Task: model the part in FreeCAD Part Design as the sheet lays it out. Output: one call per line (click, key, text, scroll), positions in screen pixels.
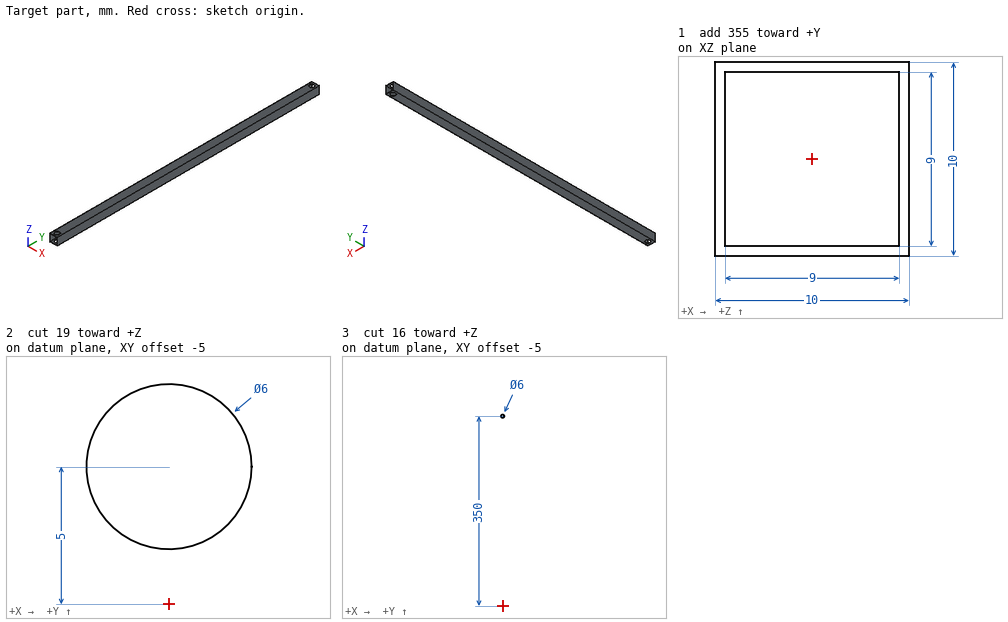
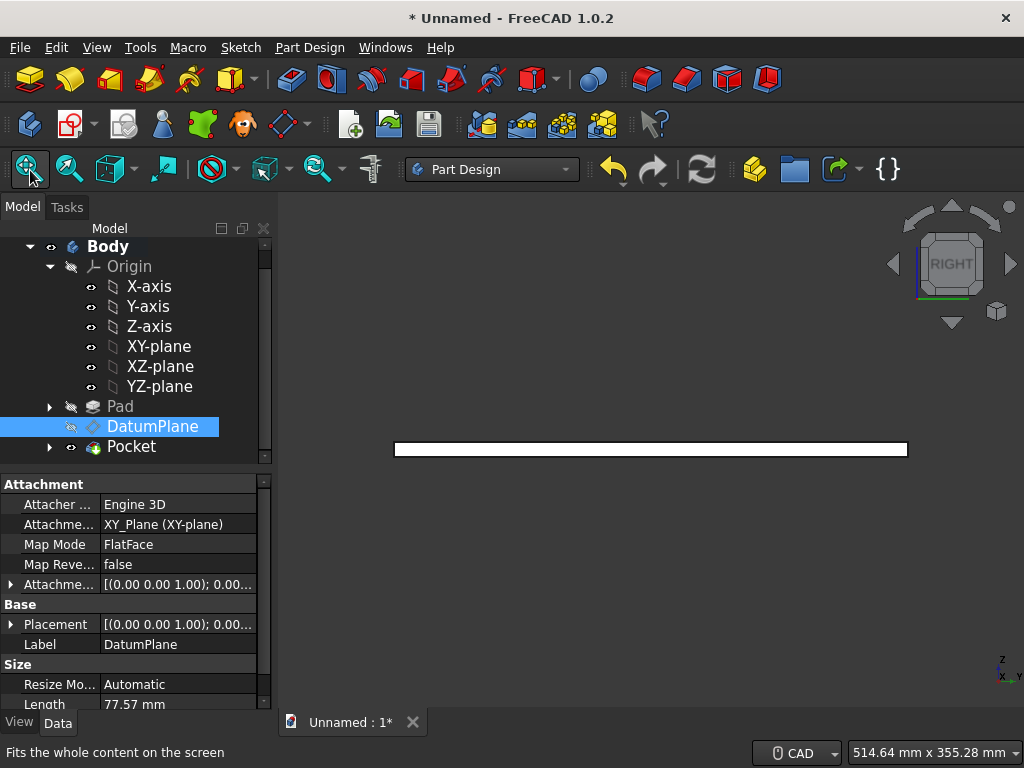
click(136, 347)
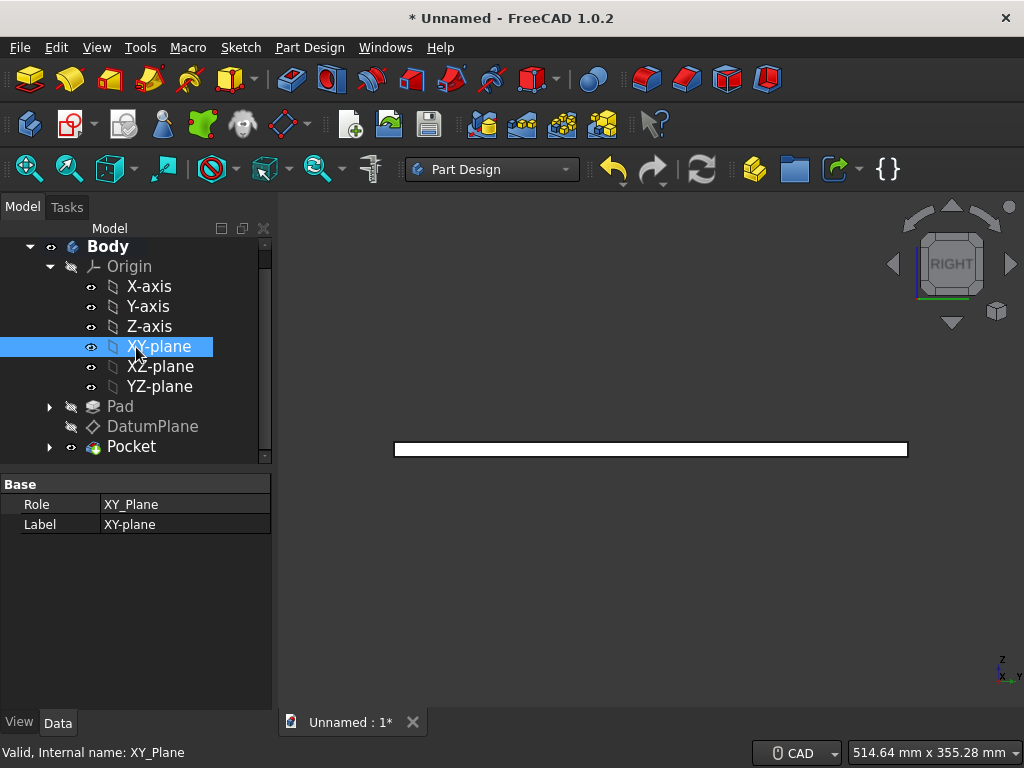
click(284, 124)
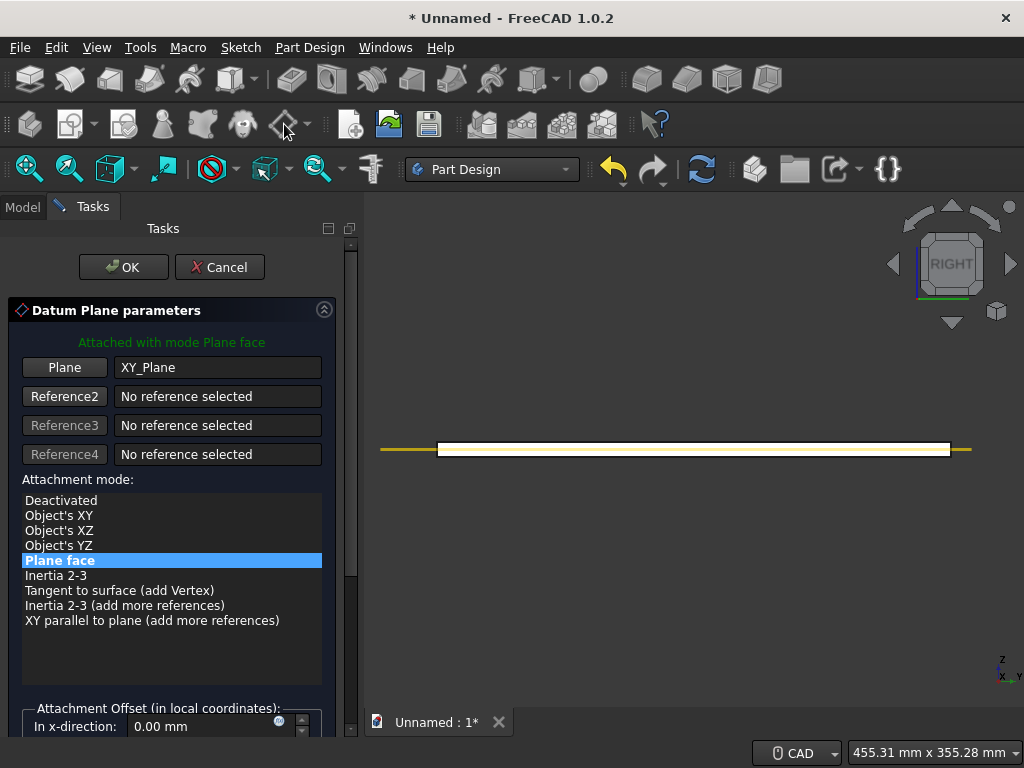
scroll(351, 487, down, 3)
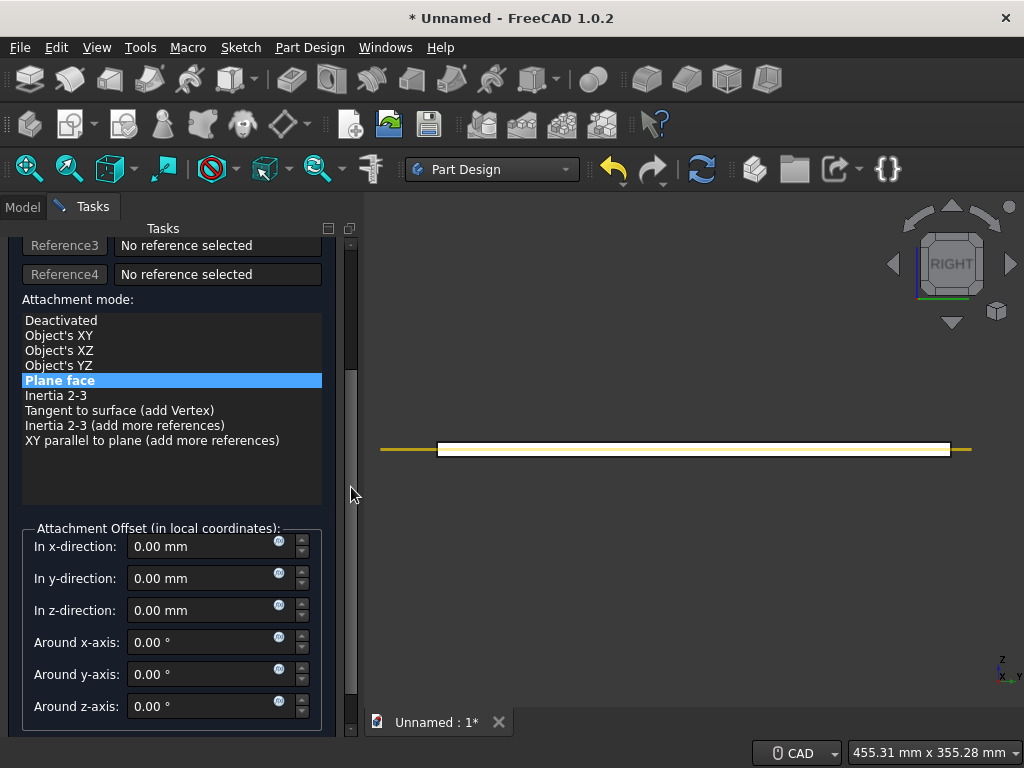
triple_click(210, 610)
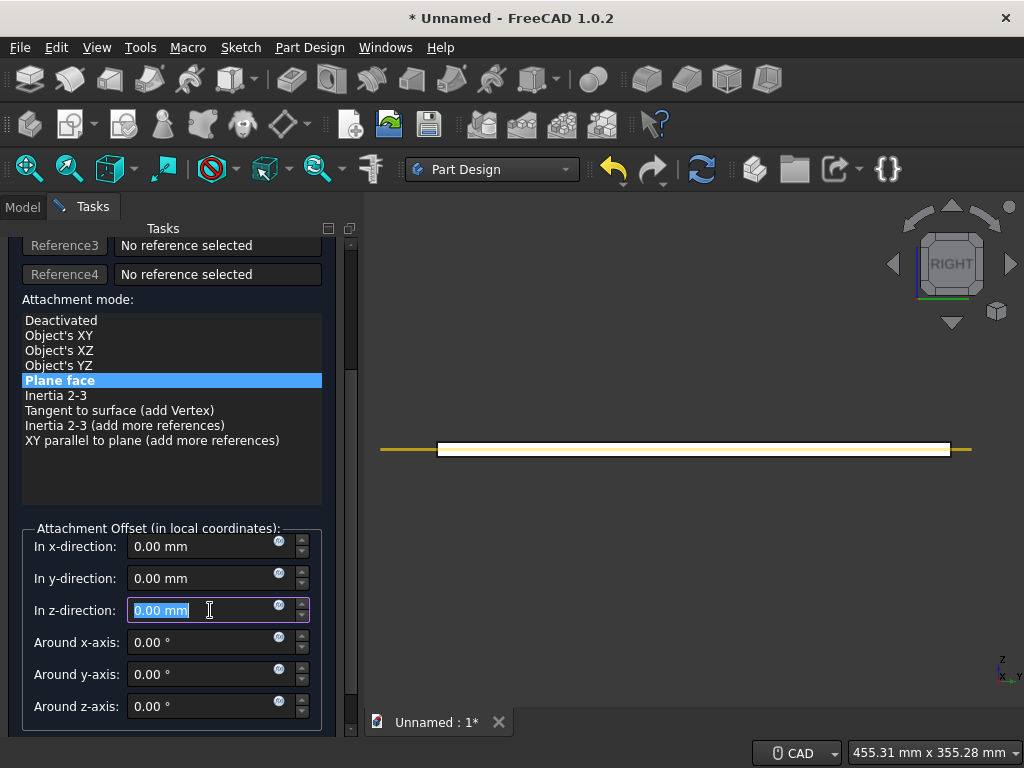
text(-5)
key(Tab)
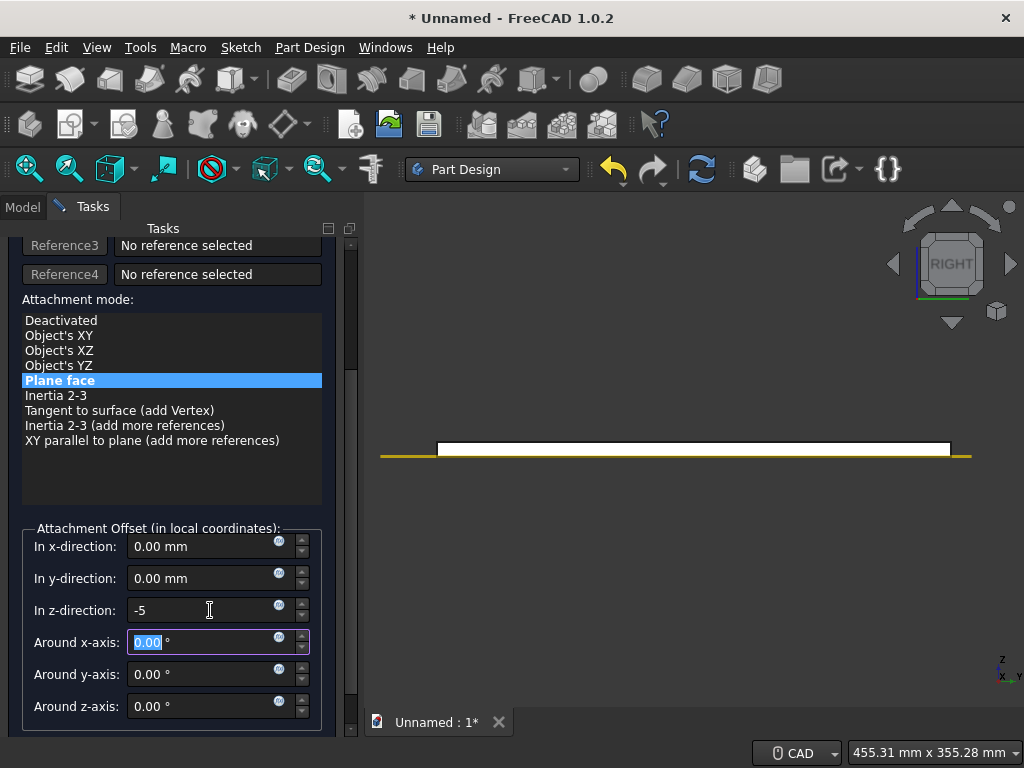
scroll(351, 487, up, 4)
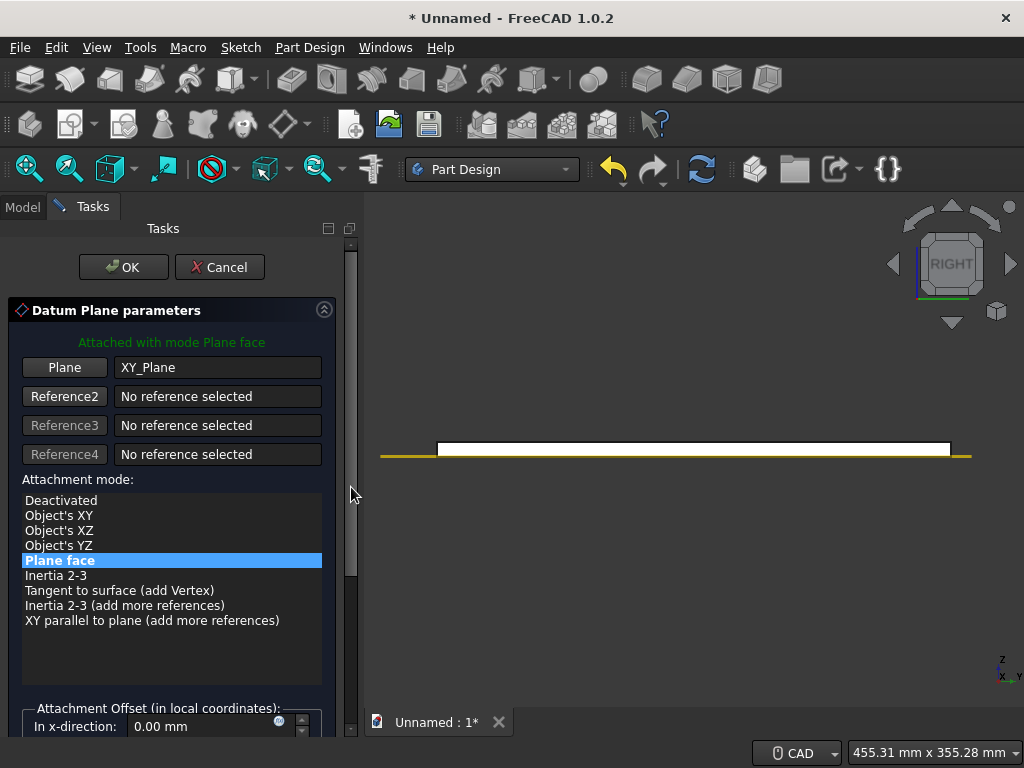
click(124, 267)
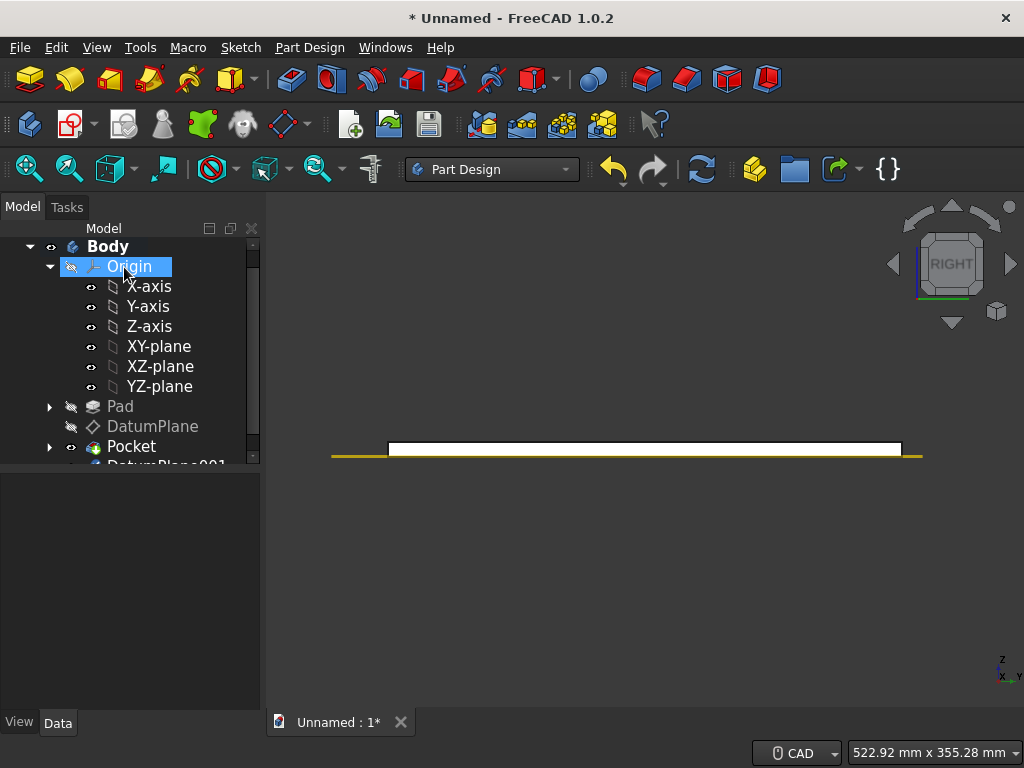
scroll(120, 342, down, 3)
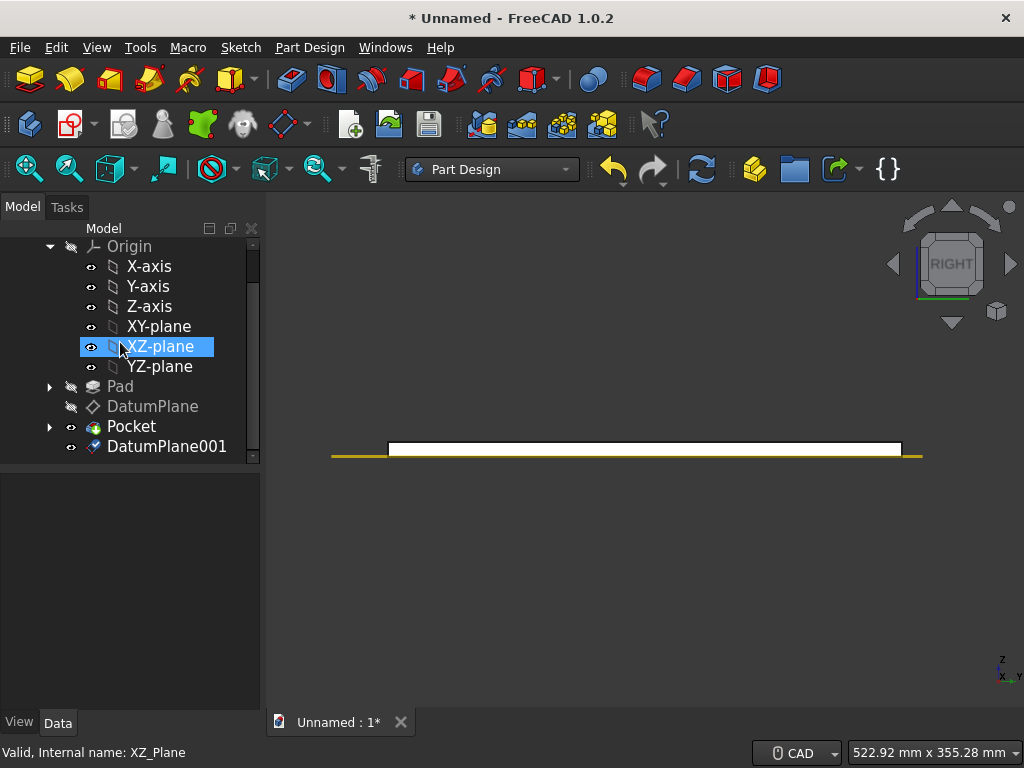
click(116, 447)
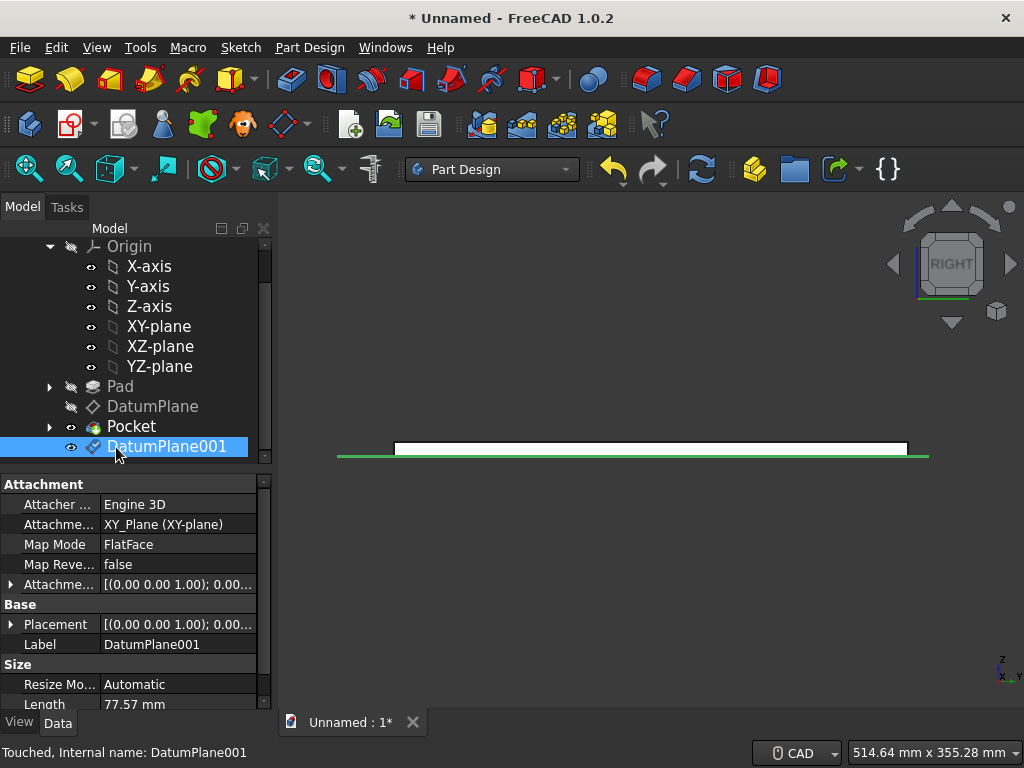
click(70, 124)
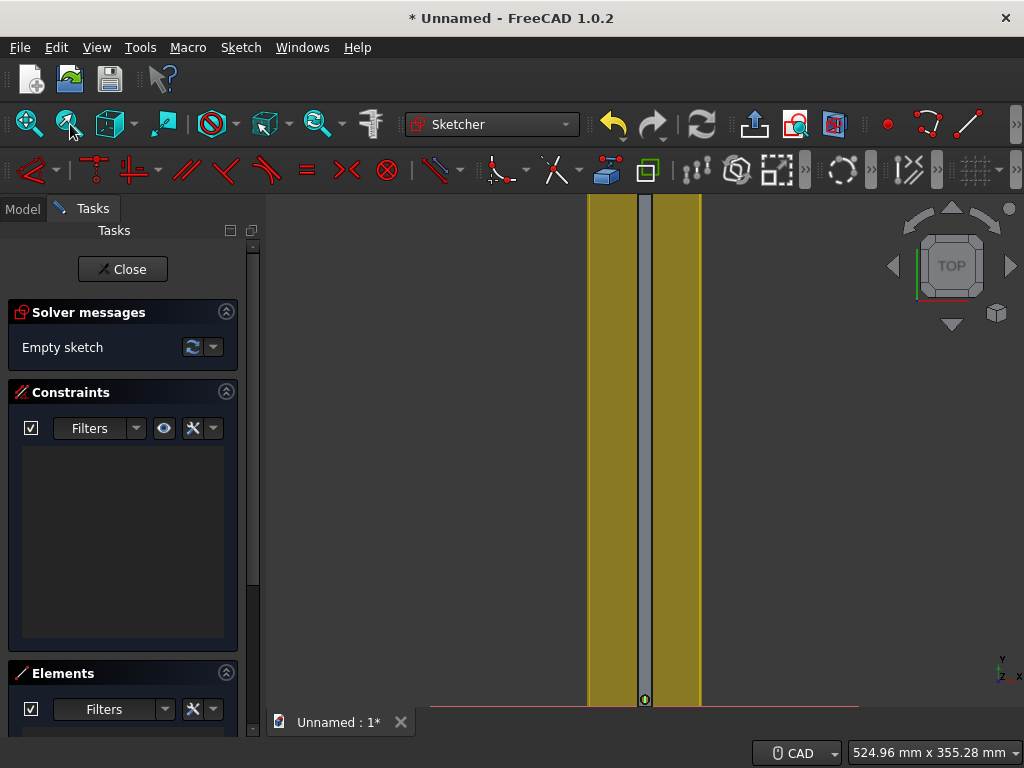
click(836, 124)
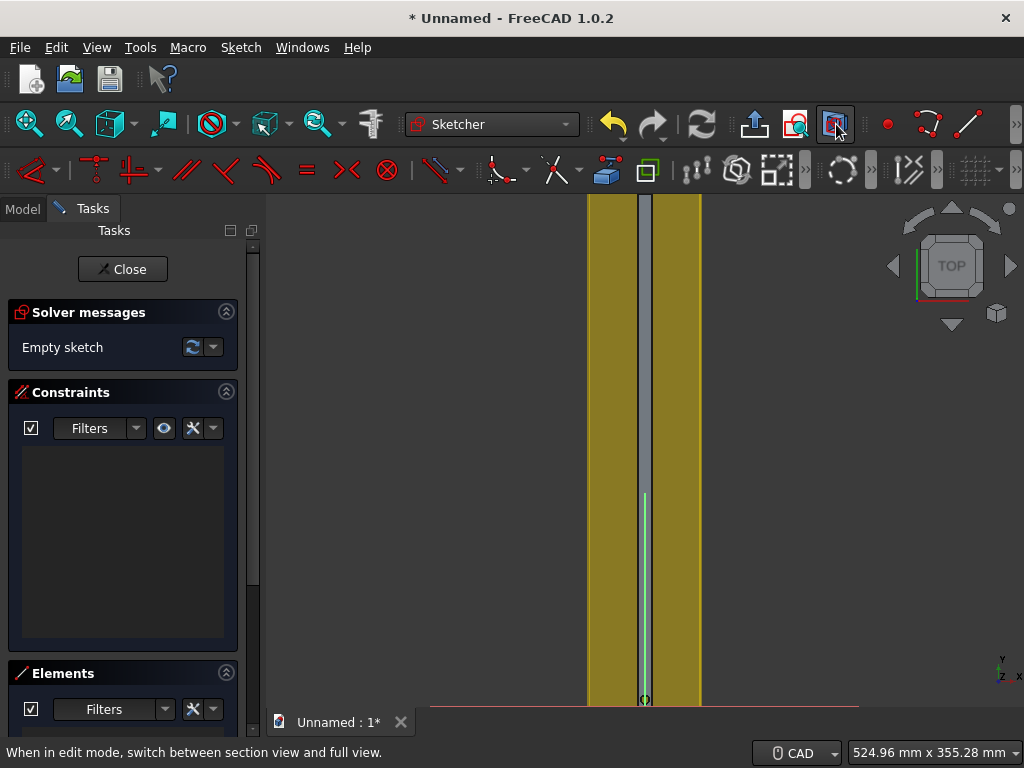
scroll(576, 450, down, 5)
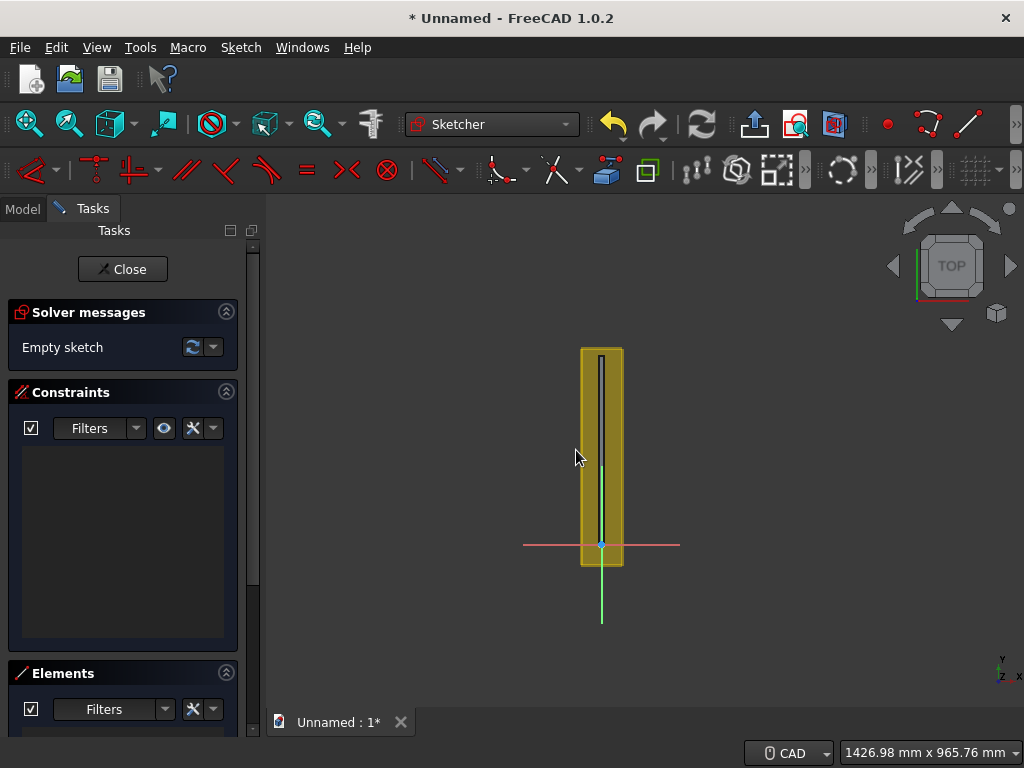
scroll(603, 354, up, 15)